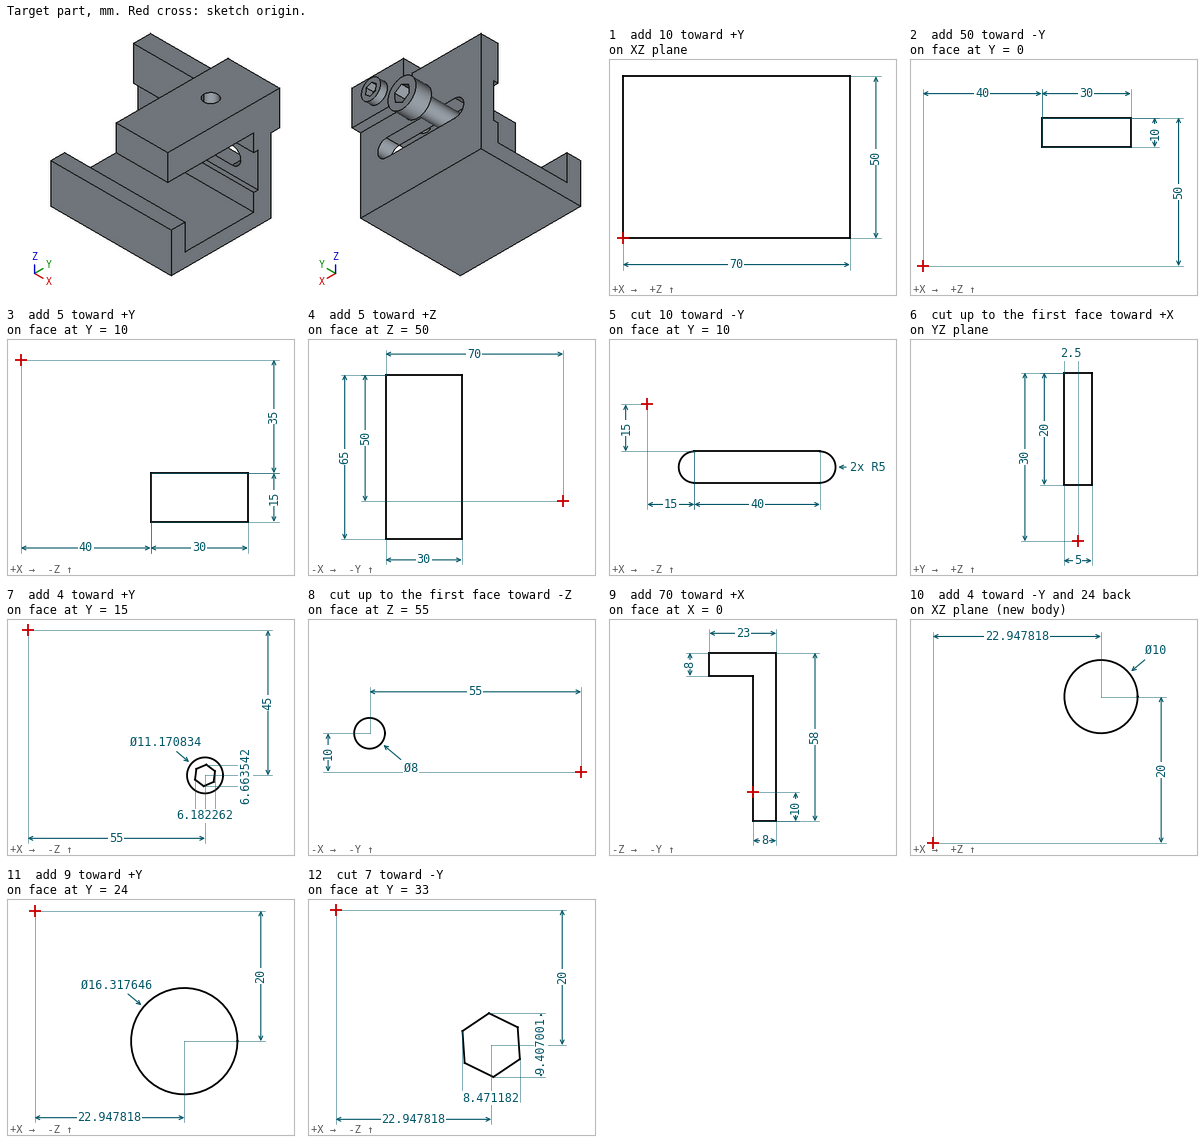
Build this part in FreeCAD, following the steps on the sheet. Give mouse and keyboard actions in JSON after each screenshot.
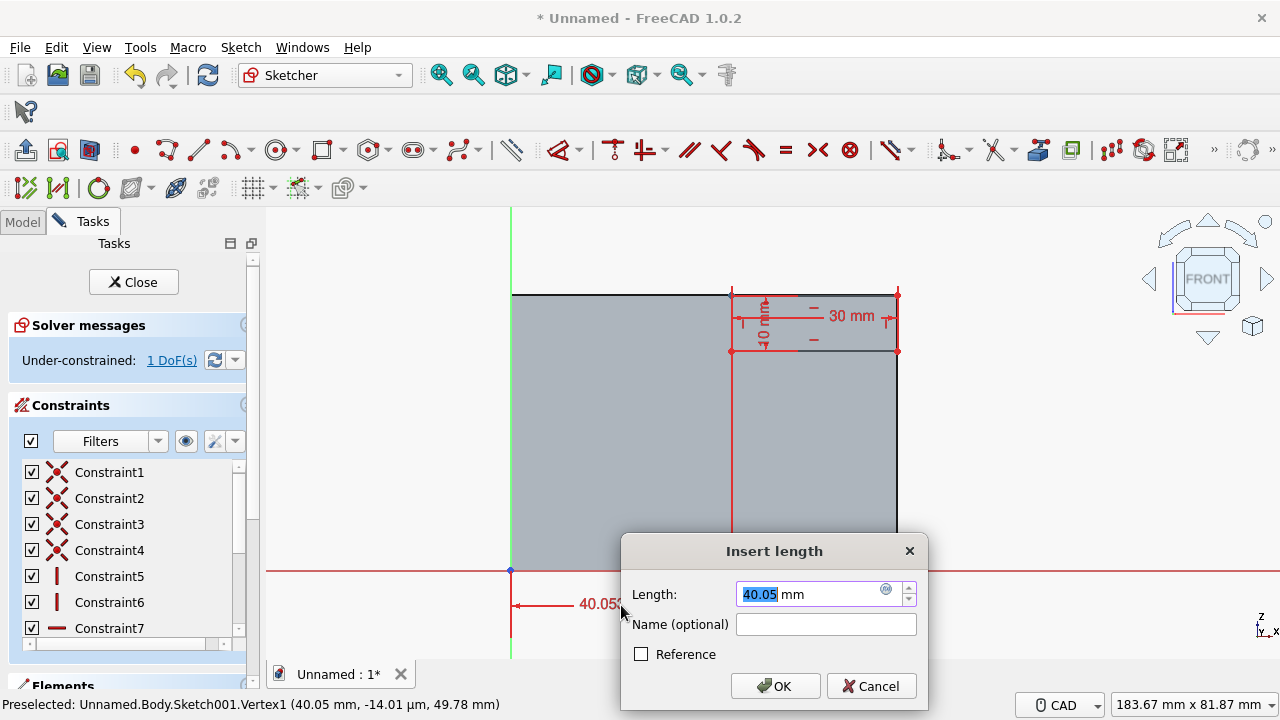
{"action": "type", "text": "40"}
{"action": "key", "text": "Return"}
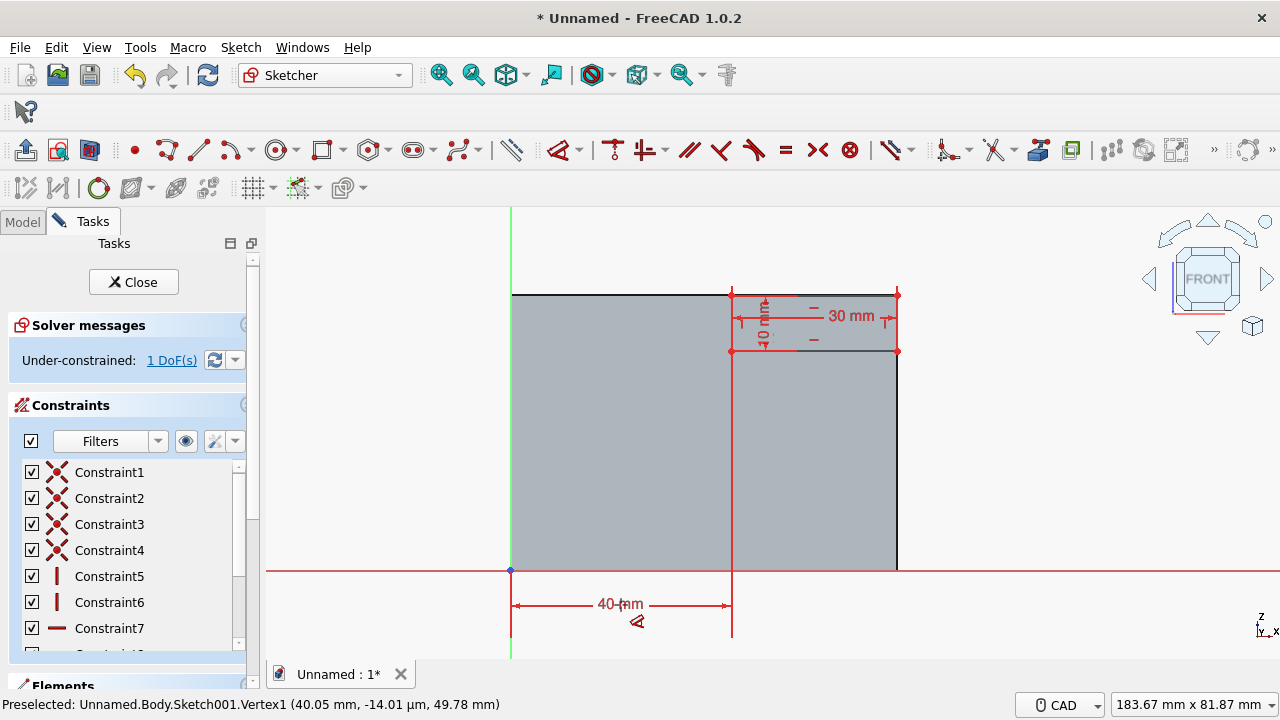
{"action": "left_click", "coordinate": [732, 296]}
{"action": "left_click", "coordinate": [477, 433]}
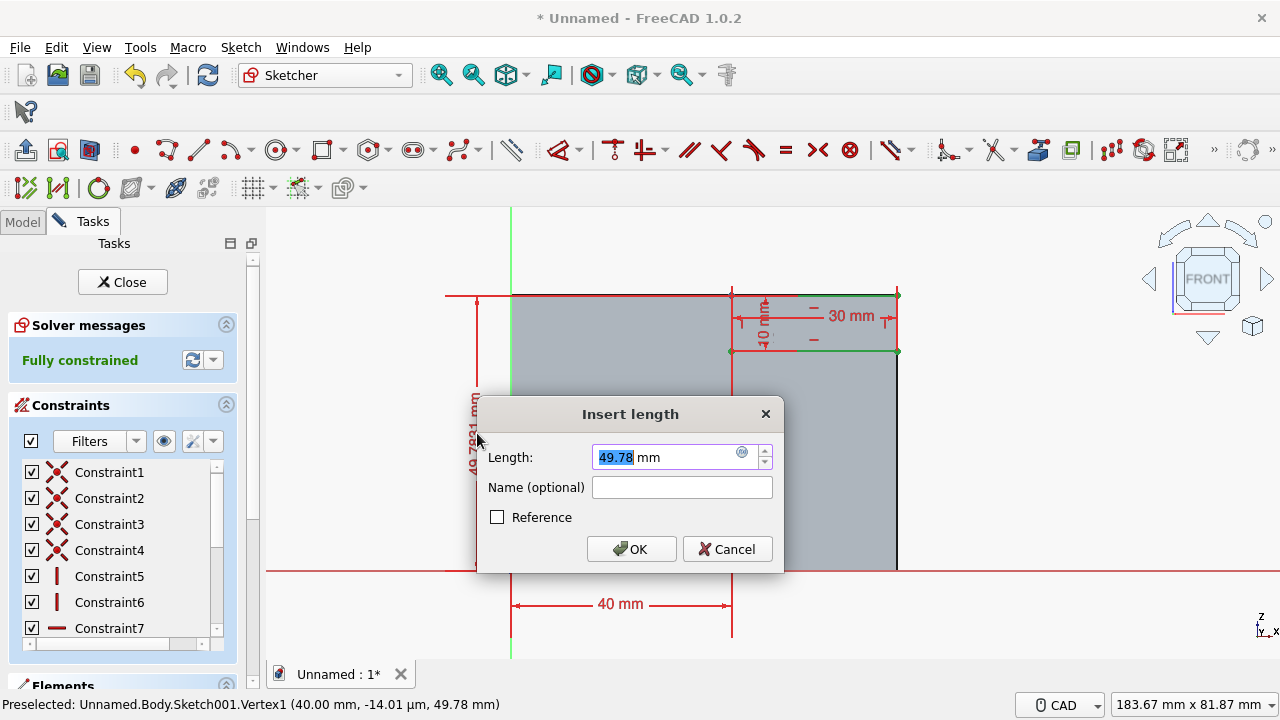
{"action": "type", "text": "50"}
{"action": "key", "text": "Return"}
{"action": "key", "text": "Escape"}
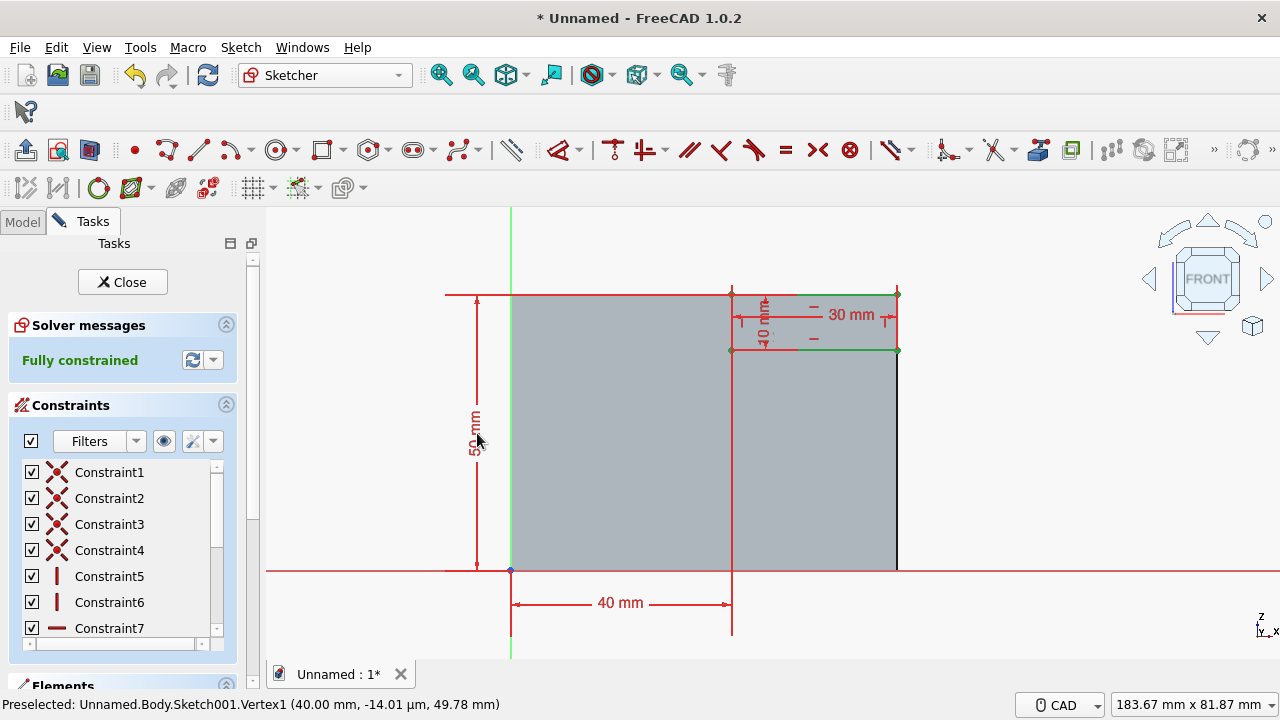
{"action": "left_click", "coordinate": [123, 282]}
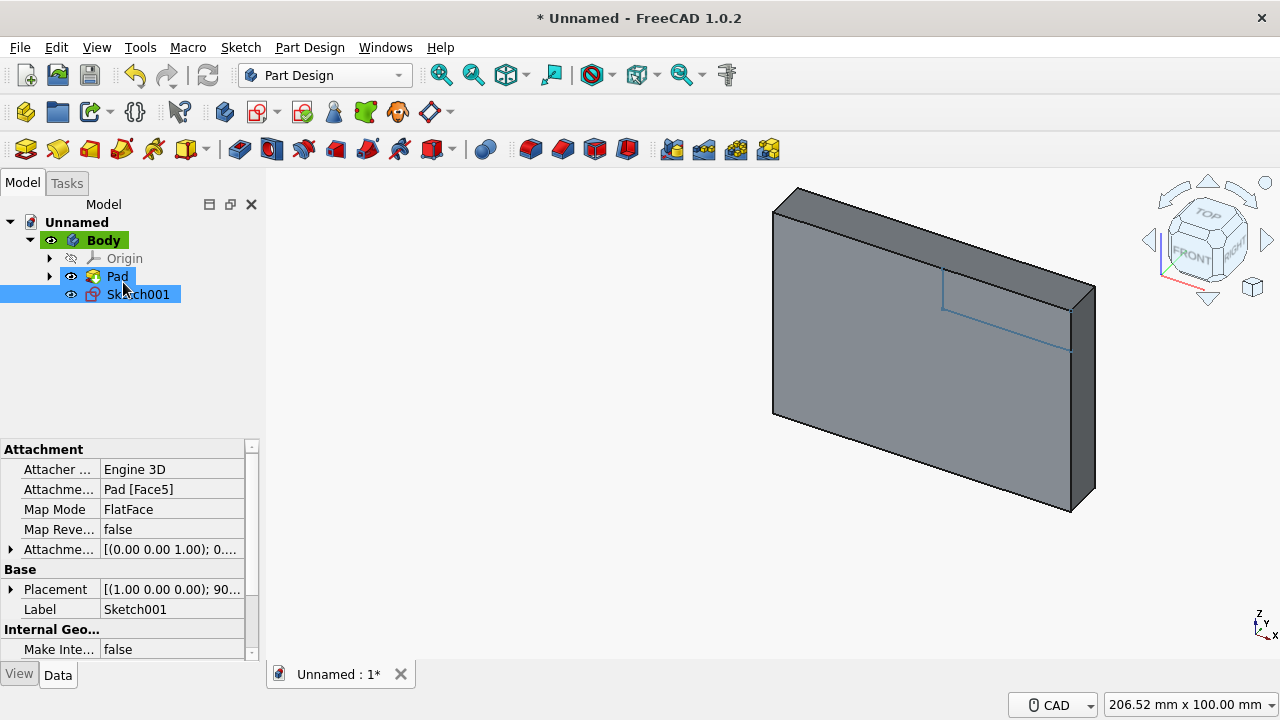
{"action": "left_click", "coordinate": [26, 150]}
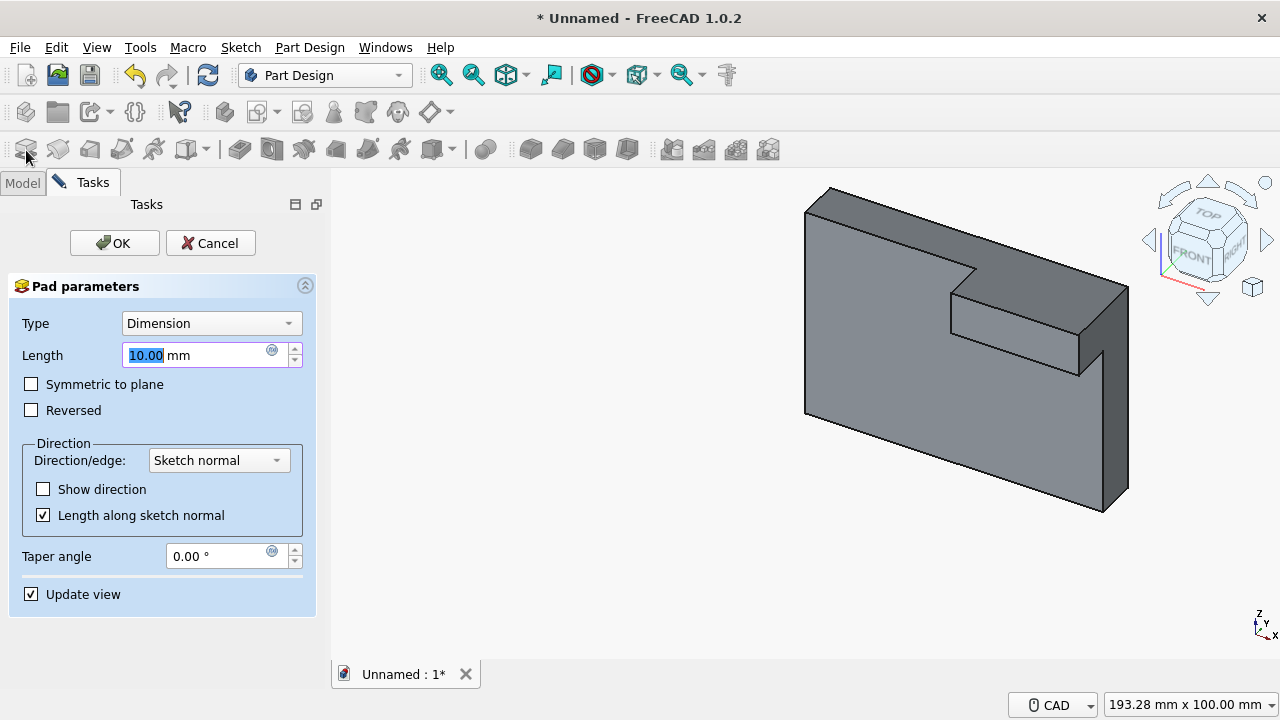
{"action": "type", "text": "50"}
{"action": "key", "text": "Tab"}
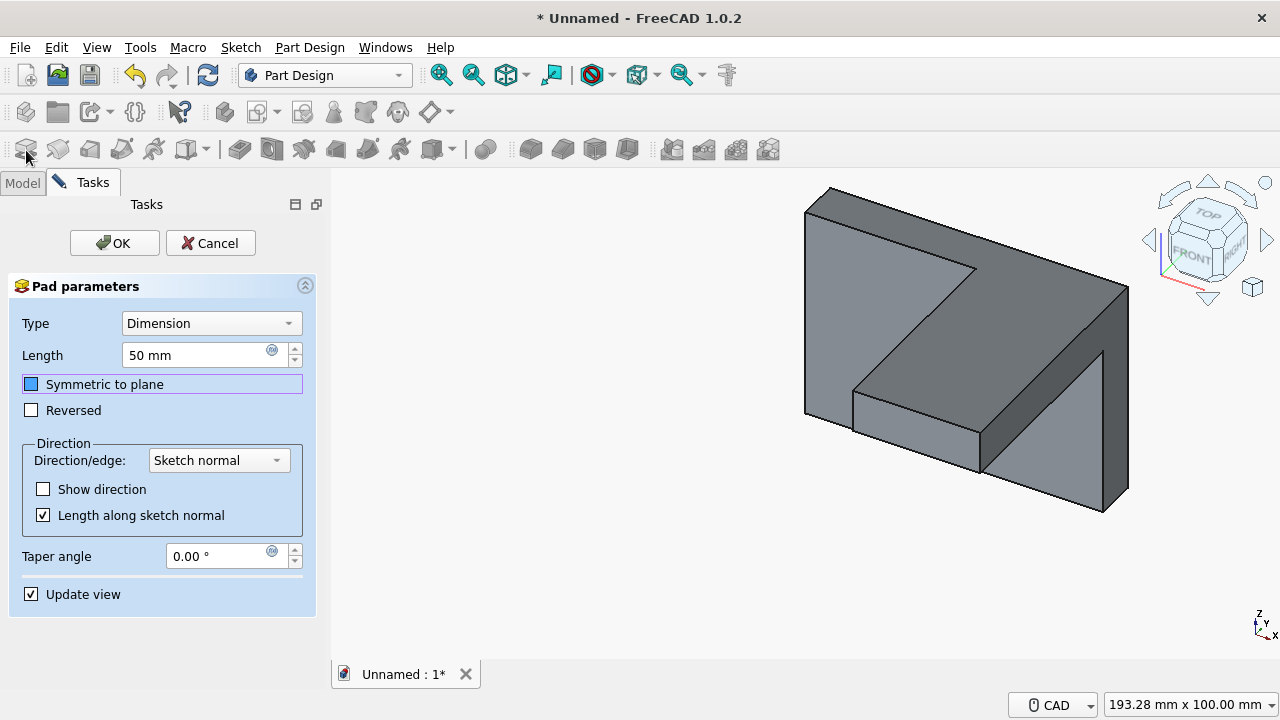
{"action": "left_click", "coordinate": [115, 243]}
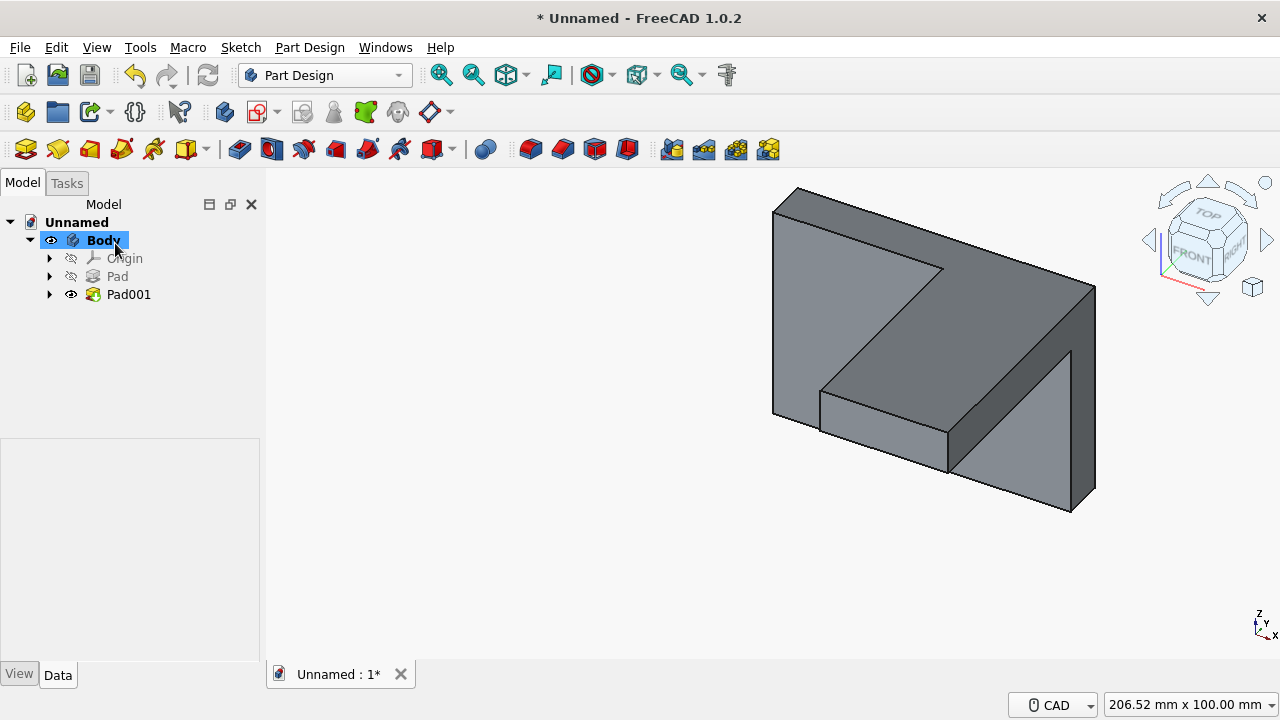
{"action": "key", "text": "4"}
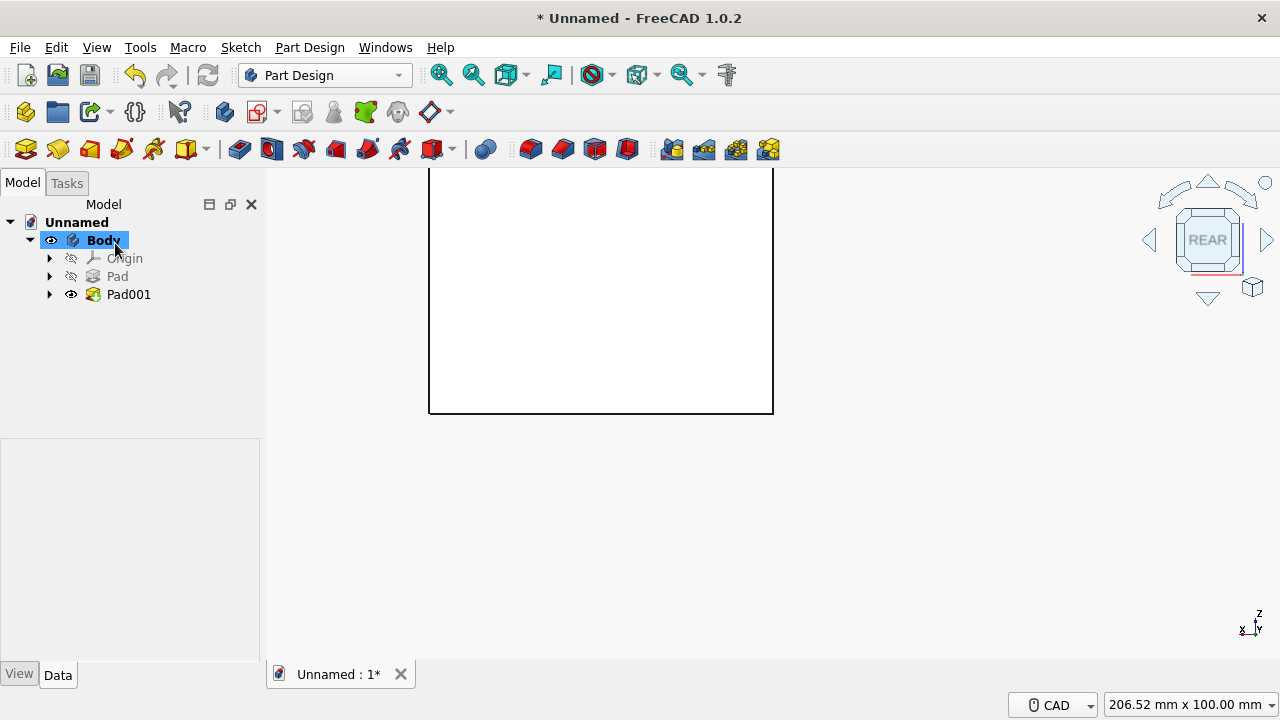
{"action": "left_click", "coordinate": [442, 76]}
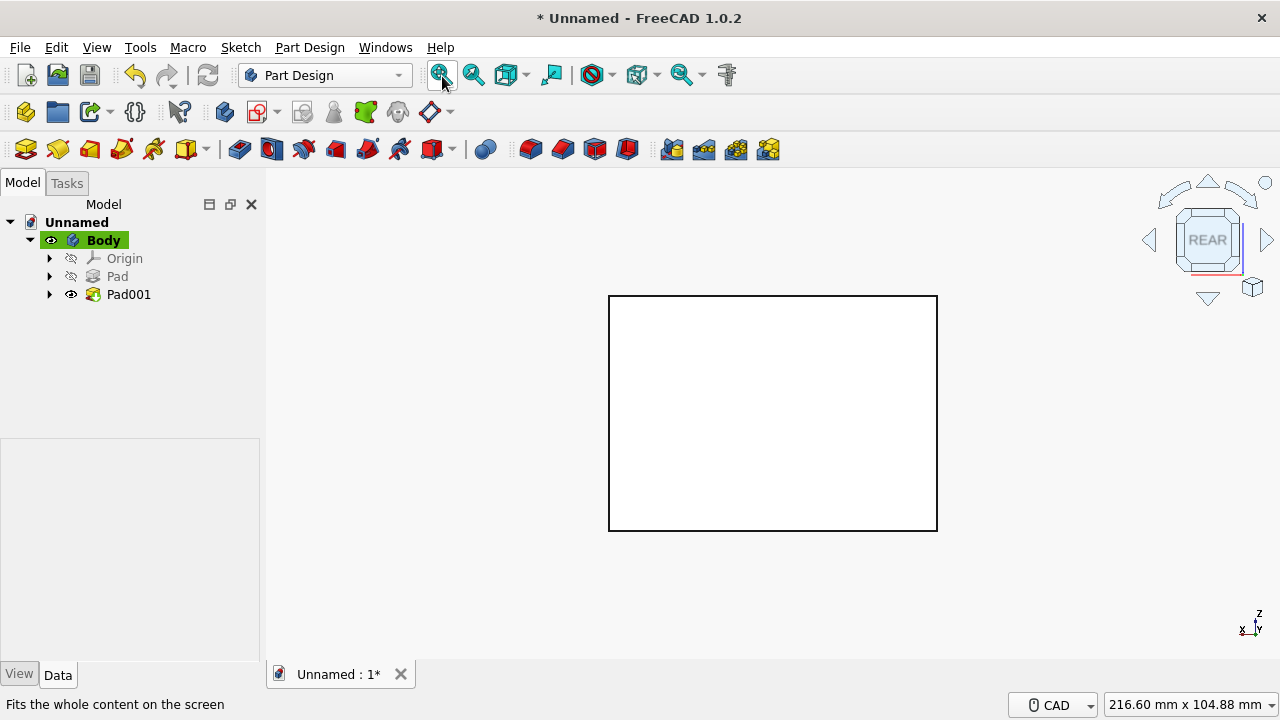
{"action": "left_click", "coordinate": [773, 413]}